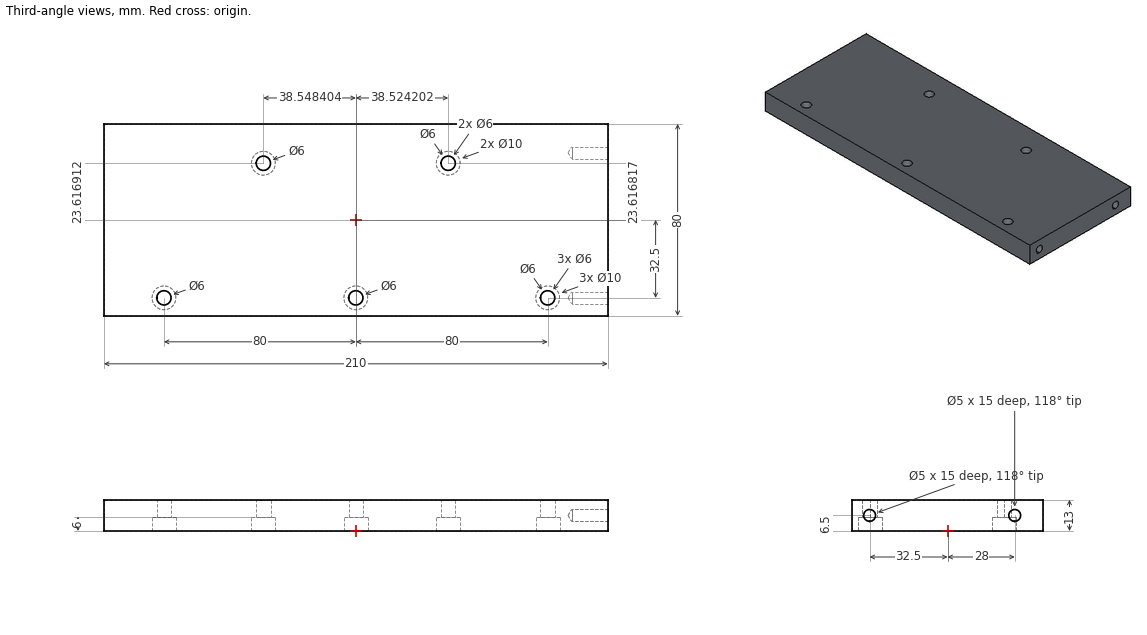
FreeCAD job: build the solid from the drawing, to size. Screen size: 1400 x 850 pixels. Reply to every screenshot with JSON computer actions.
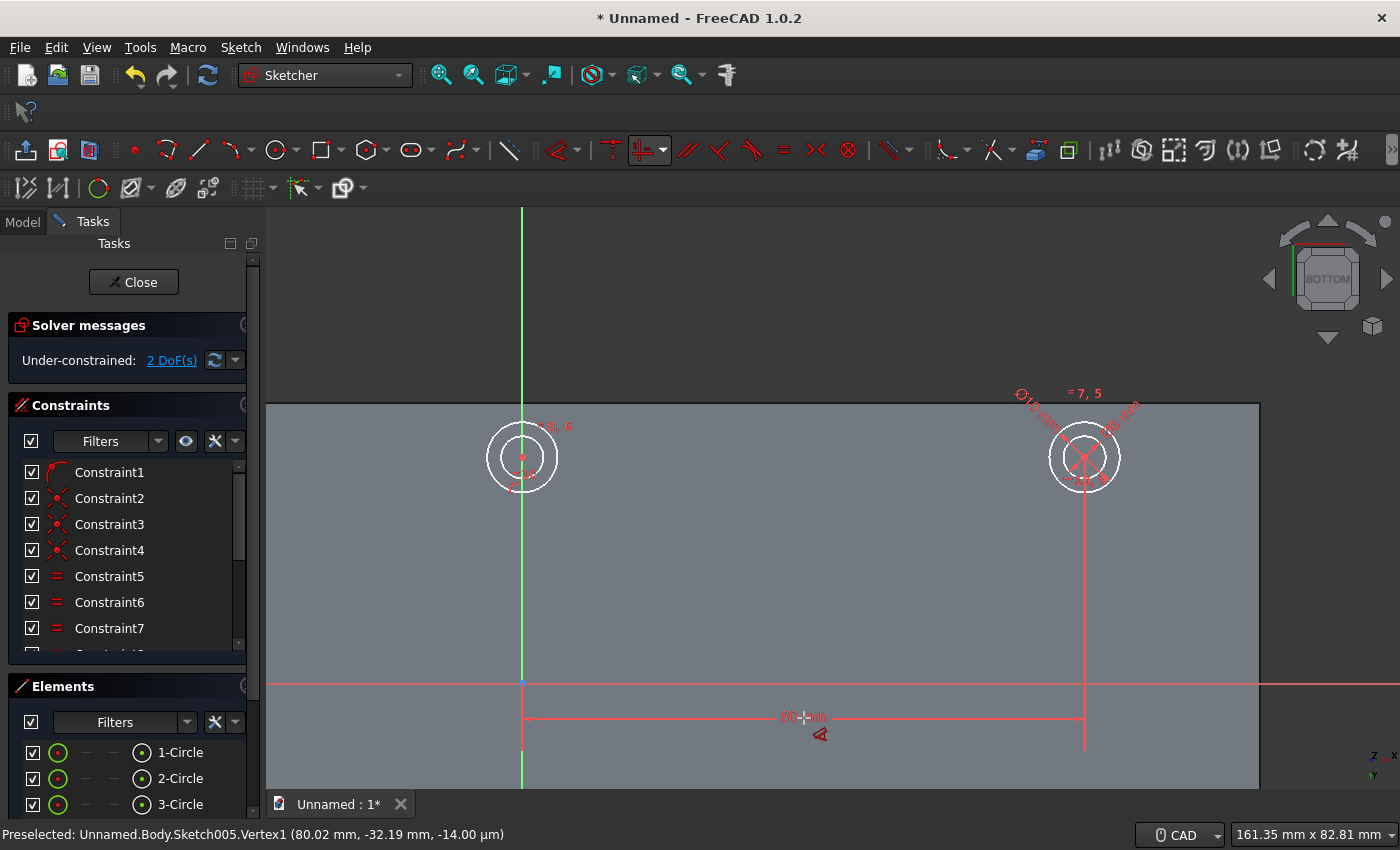
{"action": "scroll", "coordinate": [1059, 432], "scroll_direction": "down", "scroll_amount": 3}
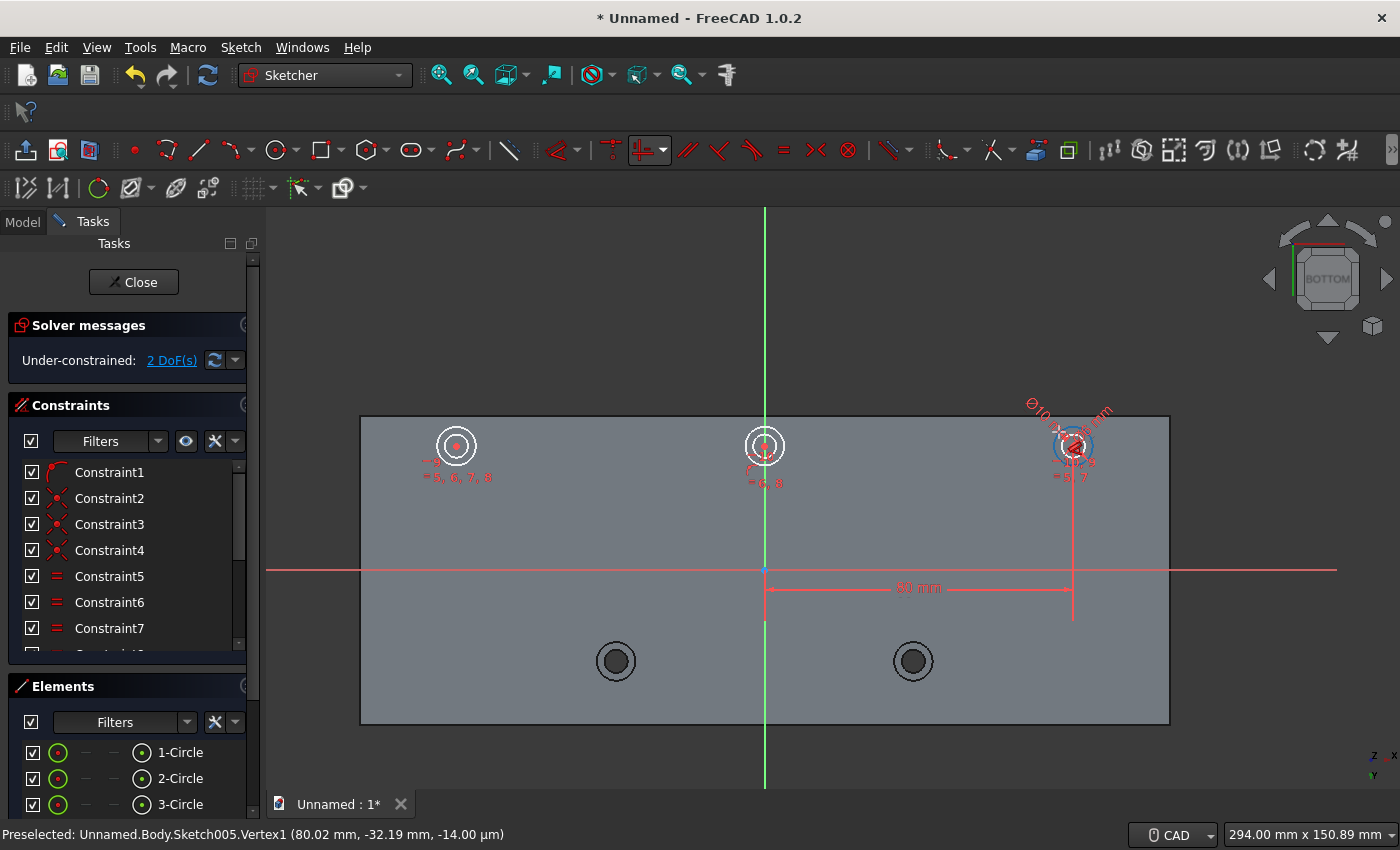
{"action": "left_click", "coordinate": [456, 446]}
{"action": "left_click", "coordinate": [611, 604]}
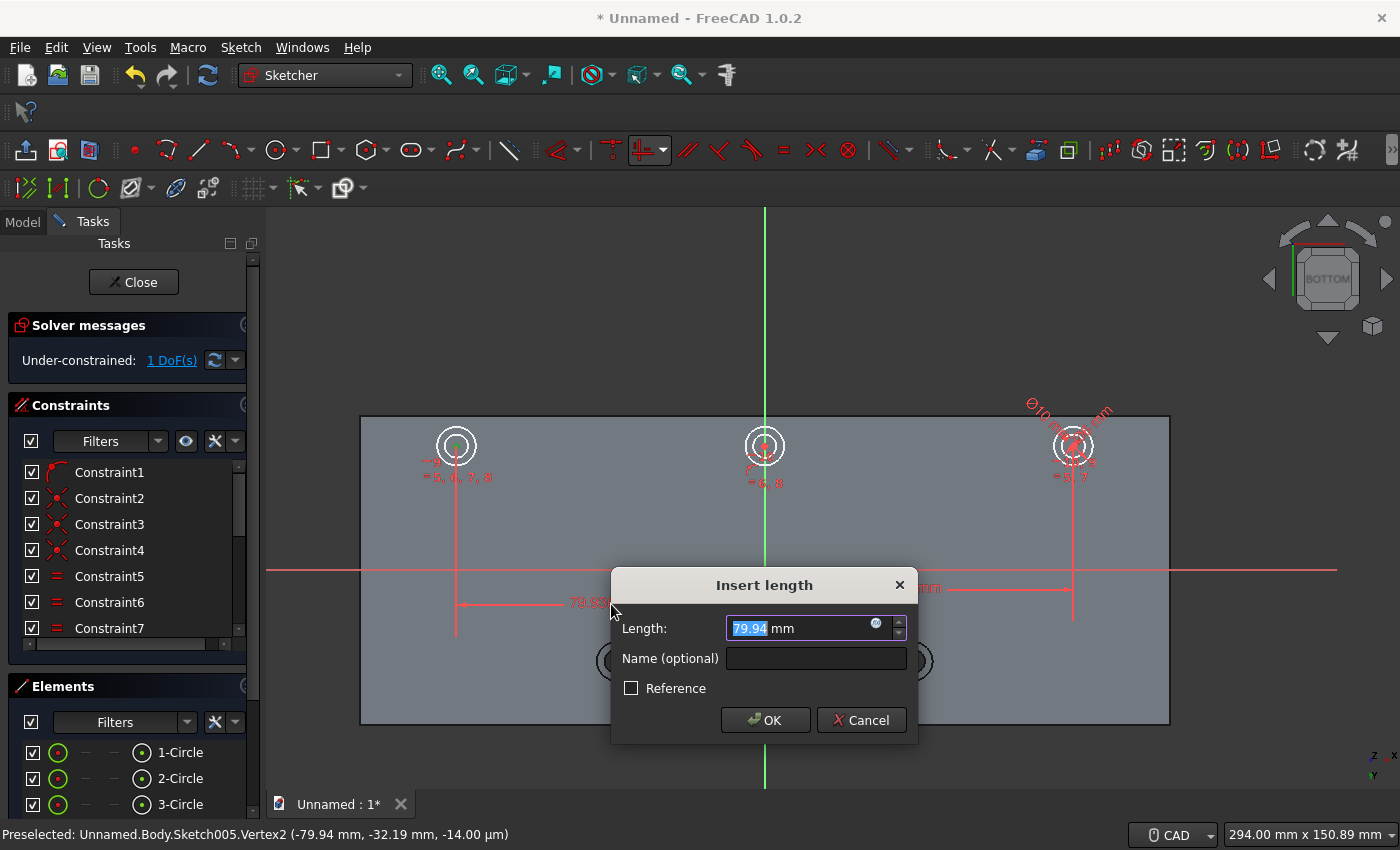
{"action": "type", "text": "80"}
{"action": "key", "text": "Return"}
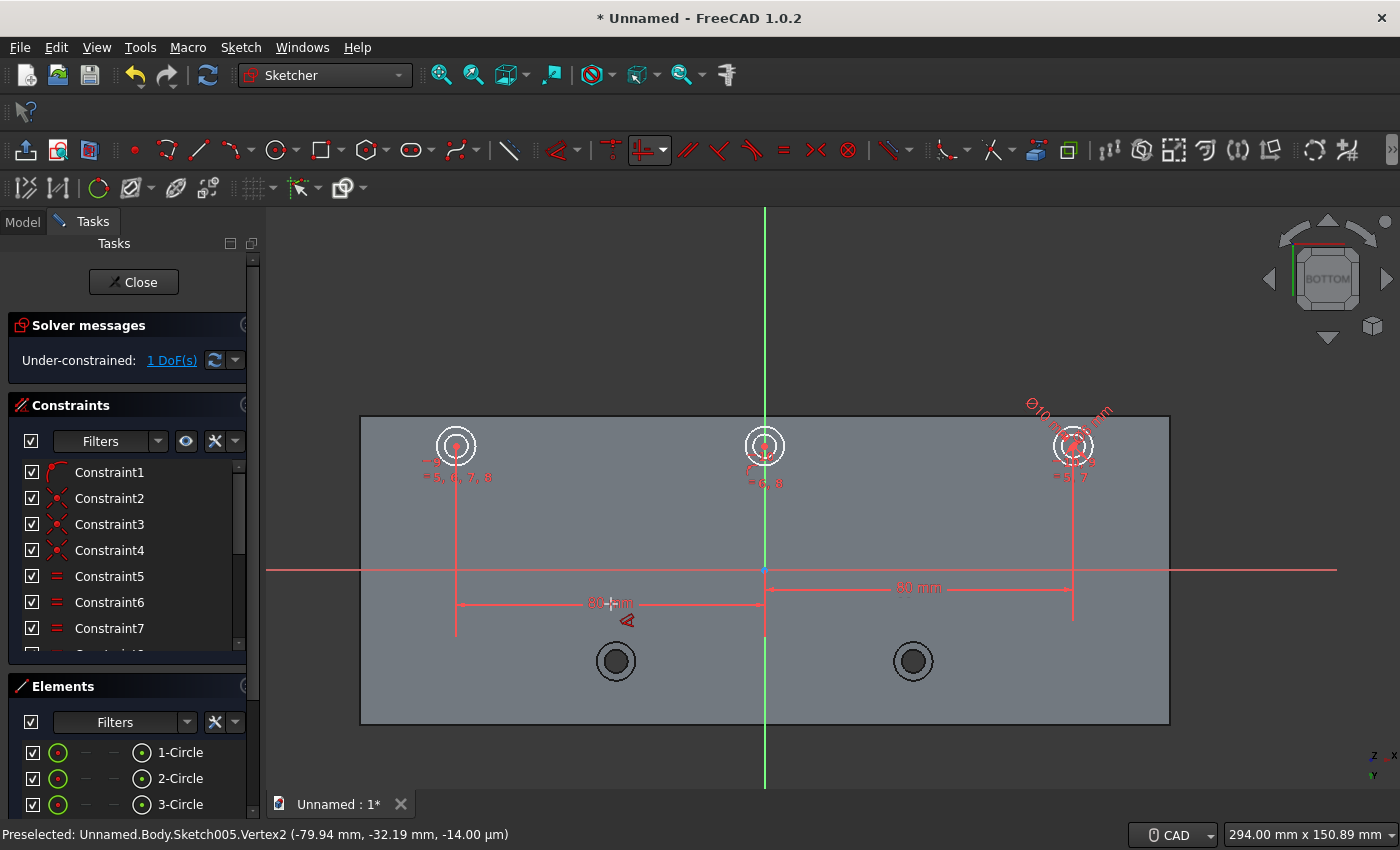
{"action": "left_click", "coordinate": [1073, 446]}
{"action": "left_click", "coordinate": [1107, 508]}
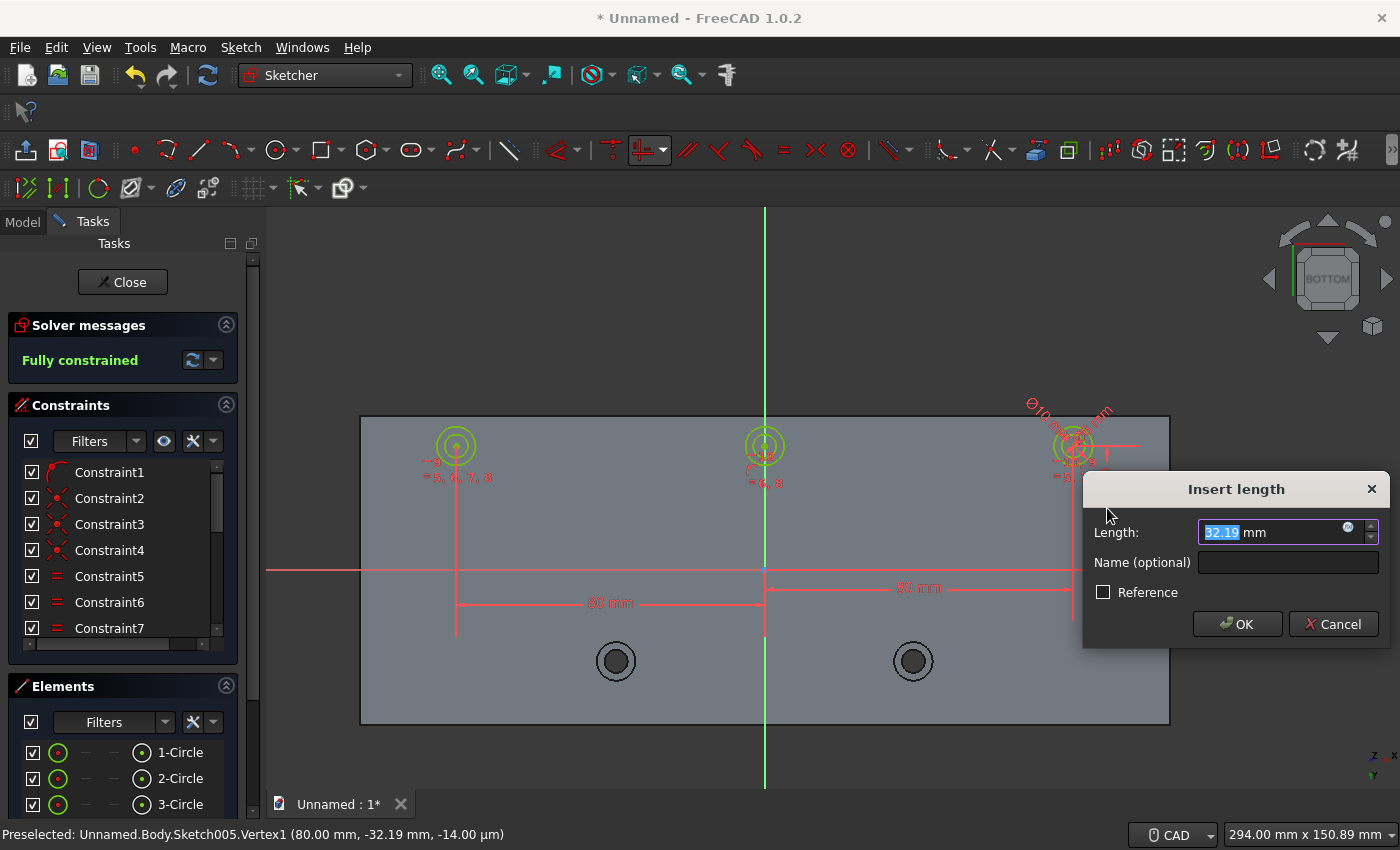
{"action": "type", "text": "32.5"}
{"action": "key", "text": "Return"}
{"action": "key", "text": "Escape"}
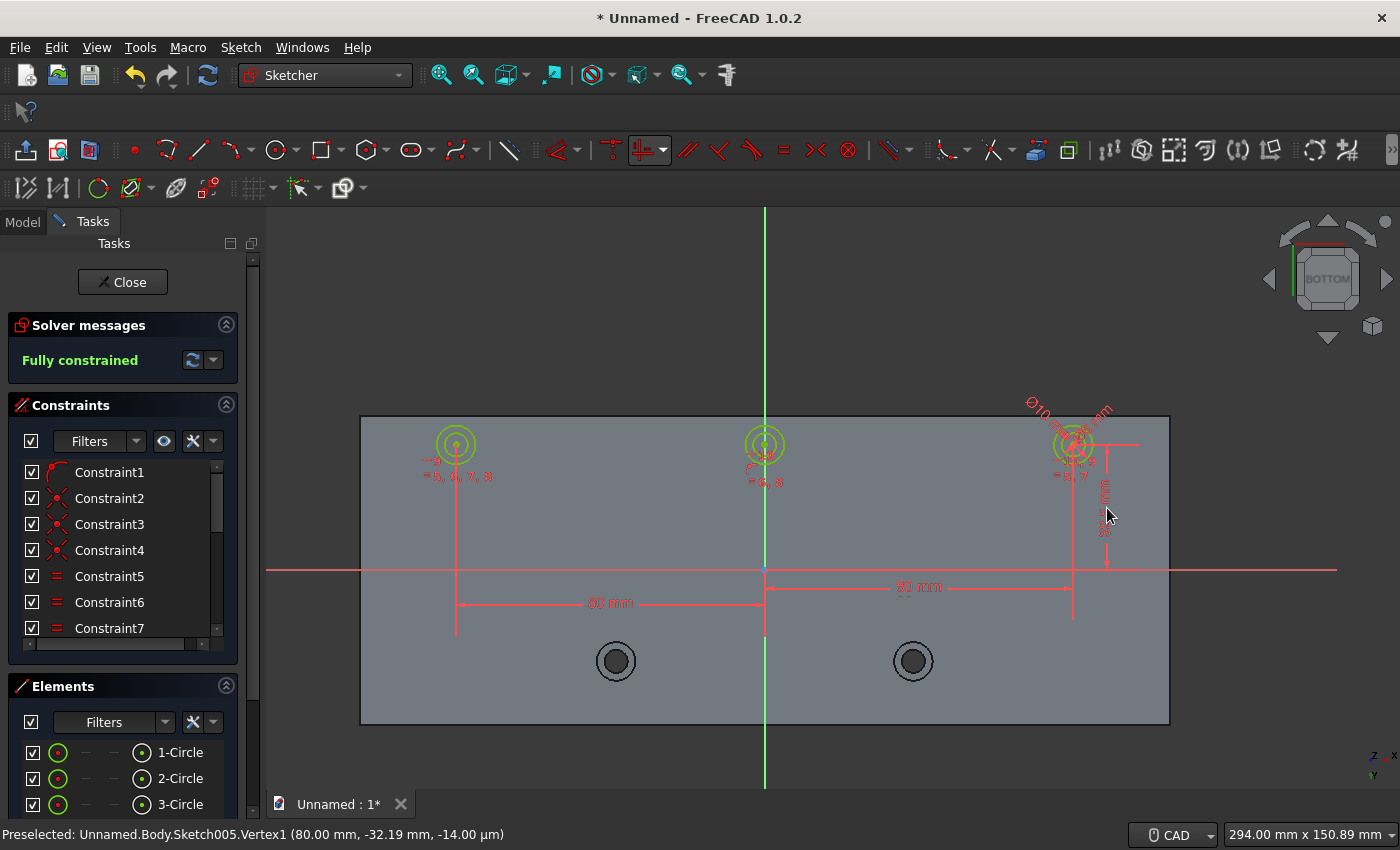
{"action": "left_click", "coordinate": [123, 282]}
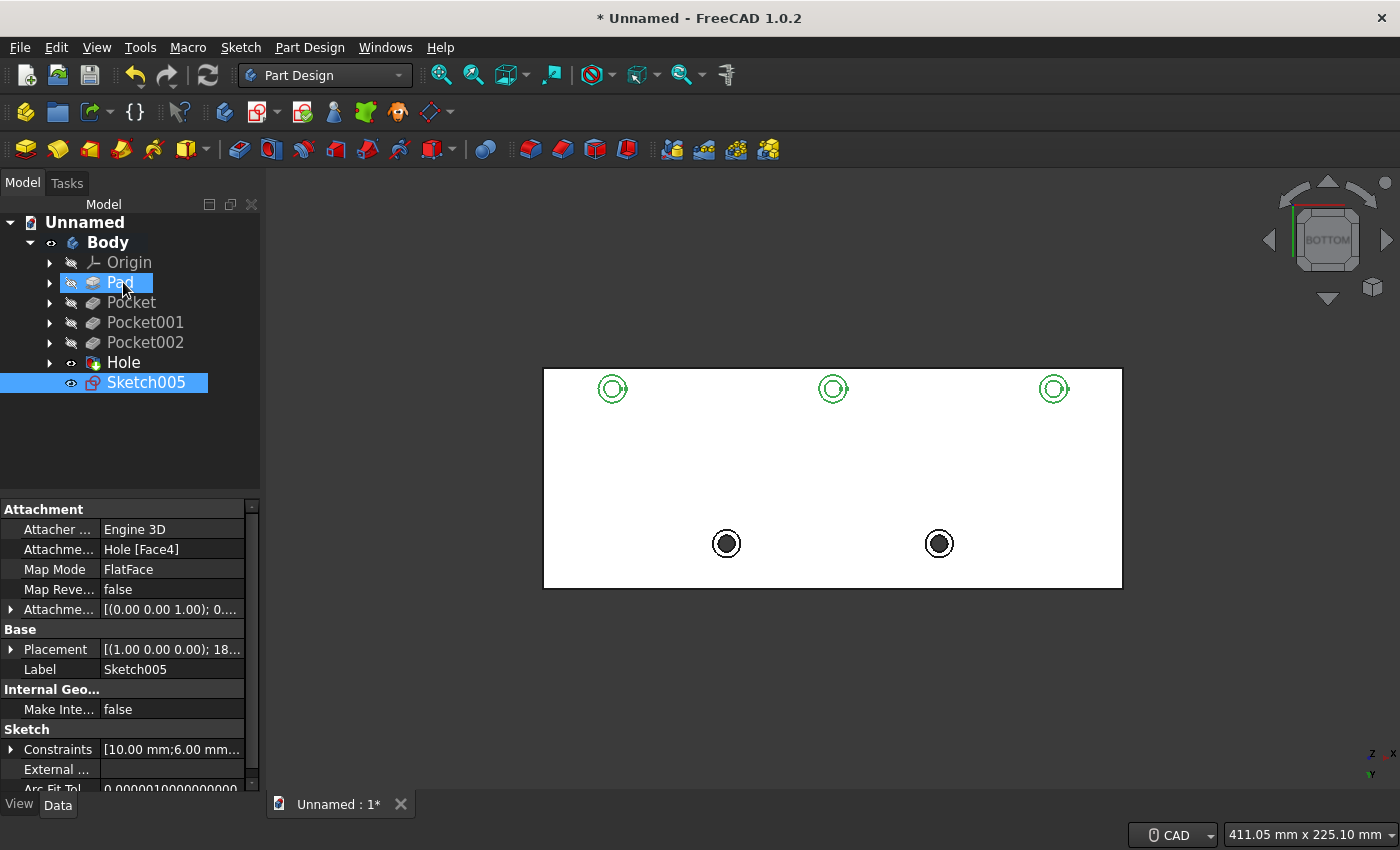
{"action": "left_click", "coordinate": [240, 150]}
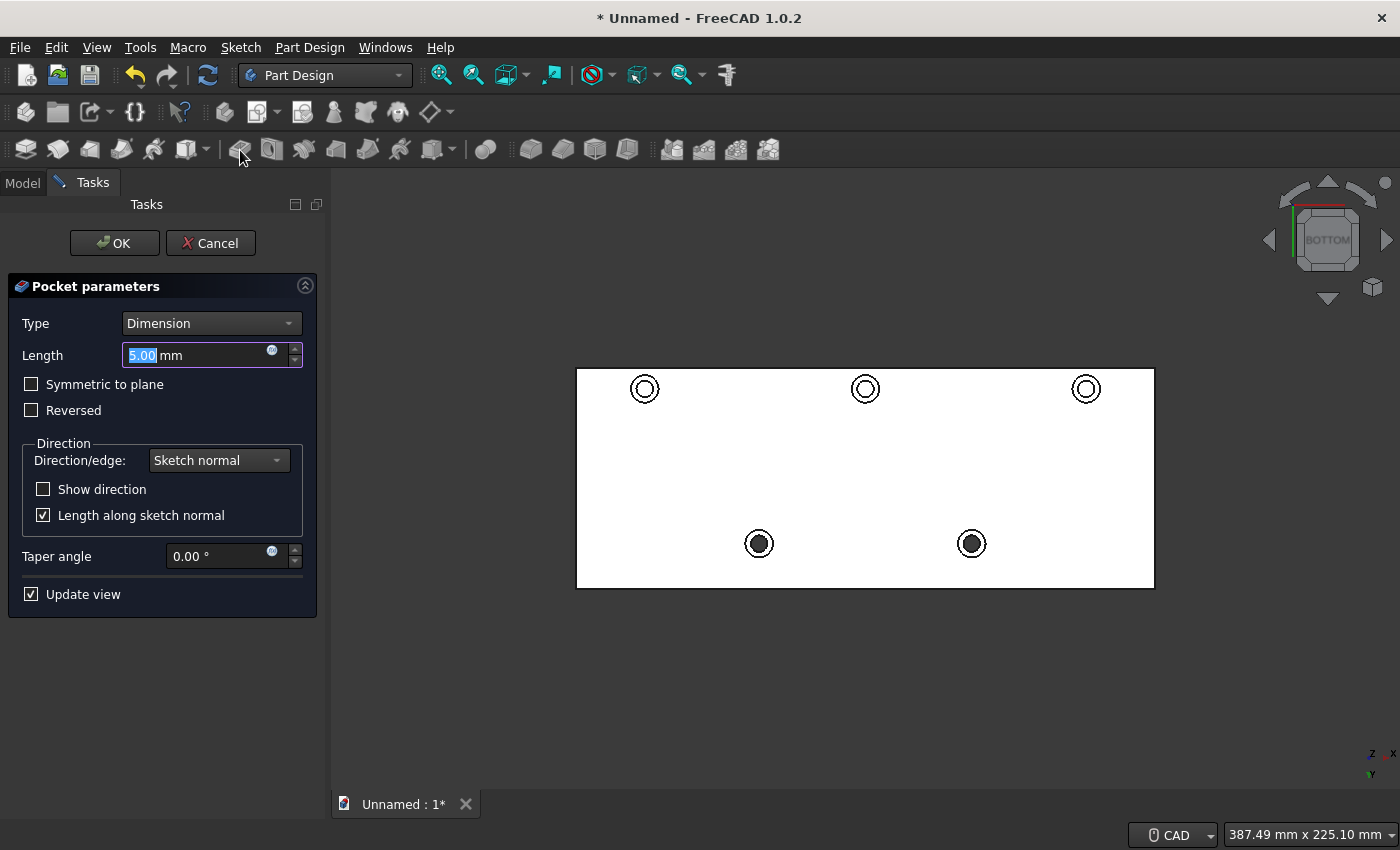
{"action": "type", "text": "6"}
{"action": "key", "text": "Tab"}